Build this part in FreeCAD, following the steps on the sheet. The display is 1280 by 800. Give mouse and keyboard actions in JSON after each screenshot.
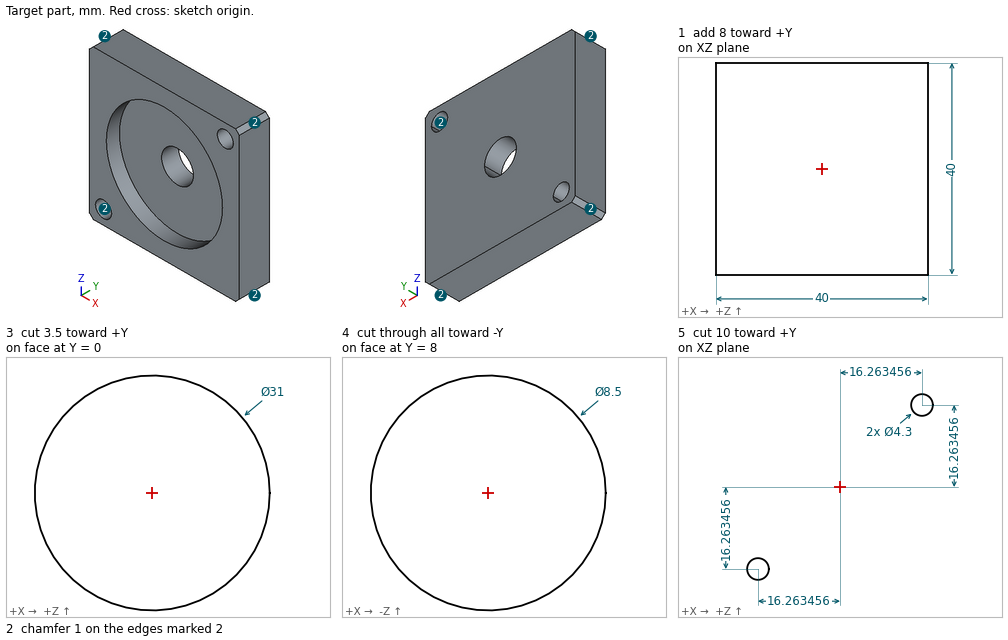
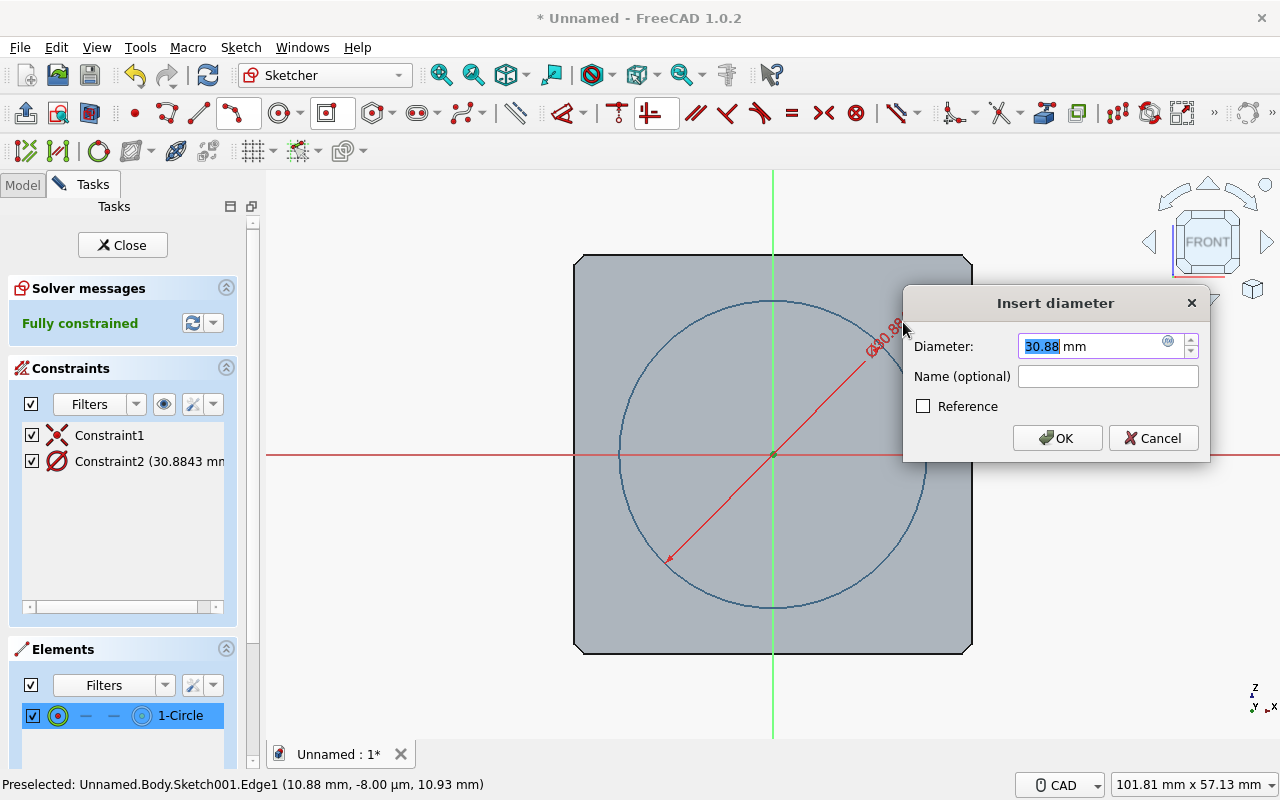
{"action": "type", "text": "31"}
{"action": "key", "text": "Return"}
{"action": "key", "text": "Escape"}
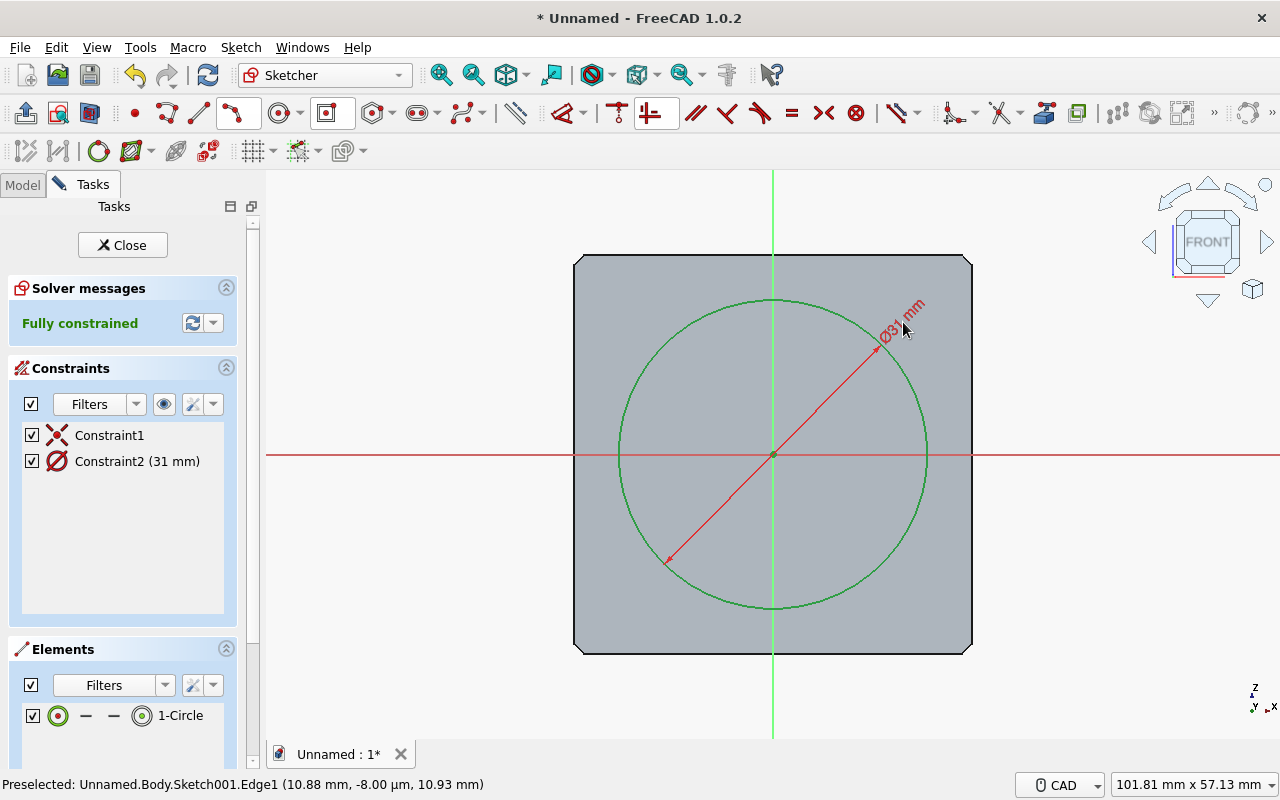
{"action": "left_click", "coordinate": [123, 245]}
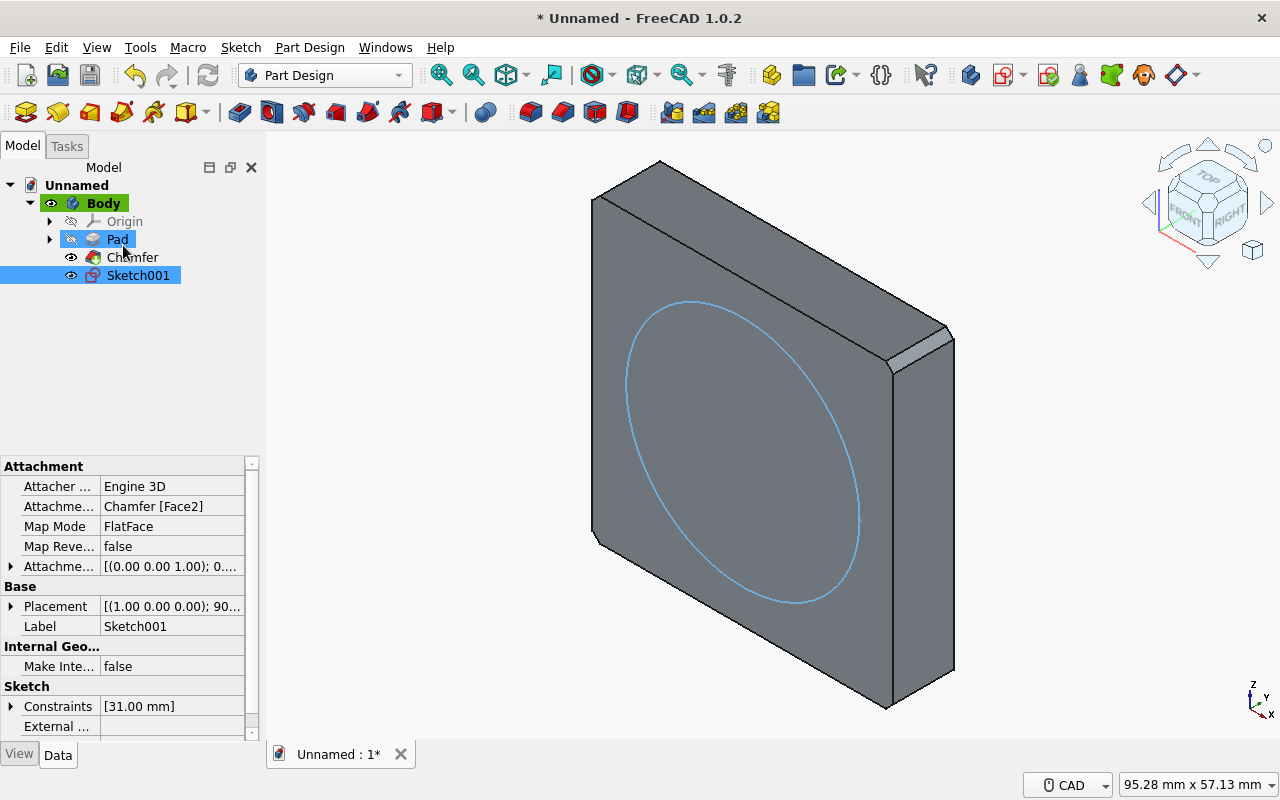
{"action": "left_click", "coordinate": [240, 112]}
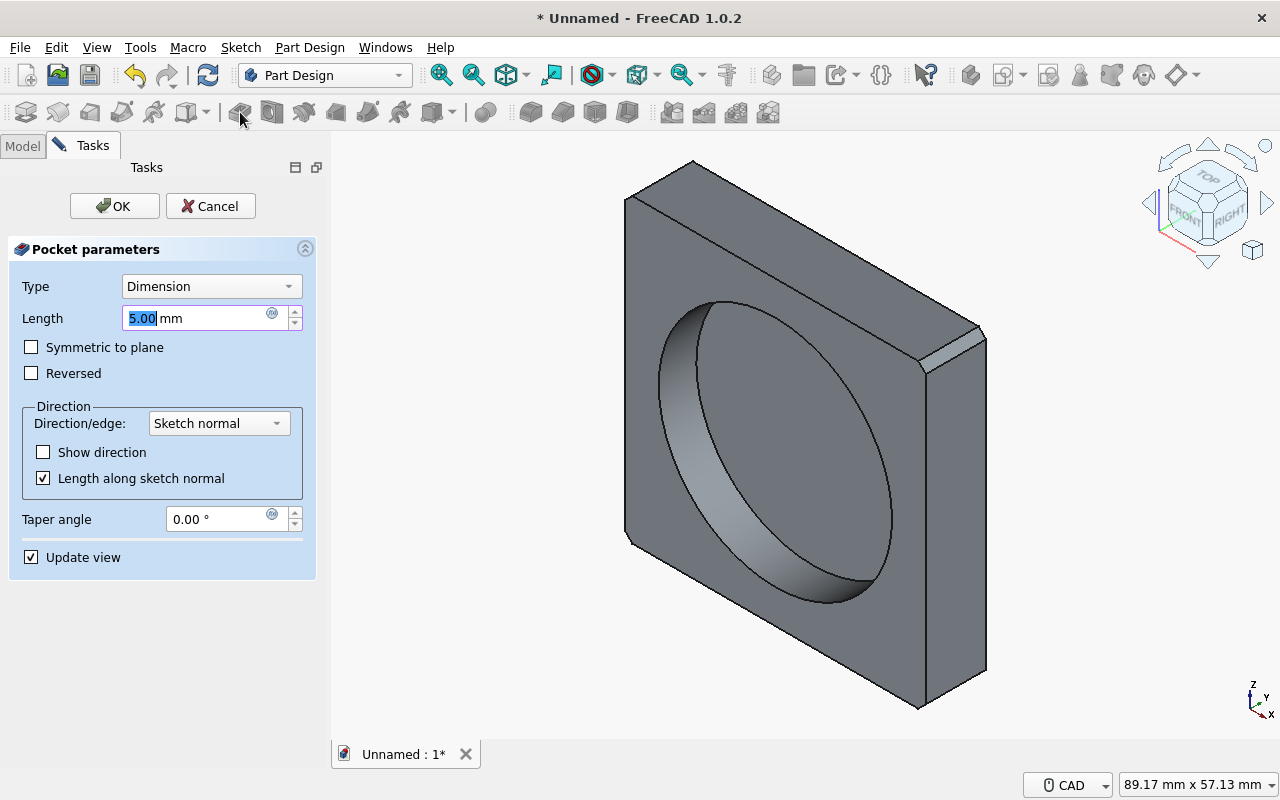
{"action": "type", "text": "3.5"}
{"action": "key", "text": "Tab"}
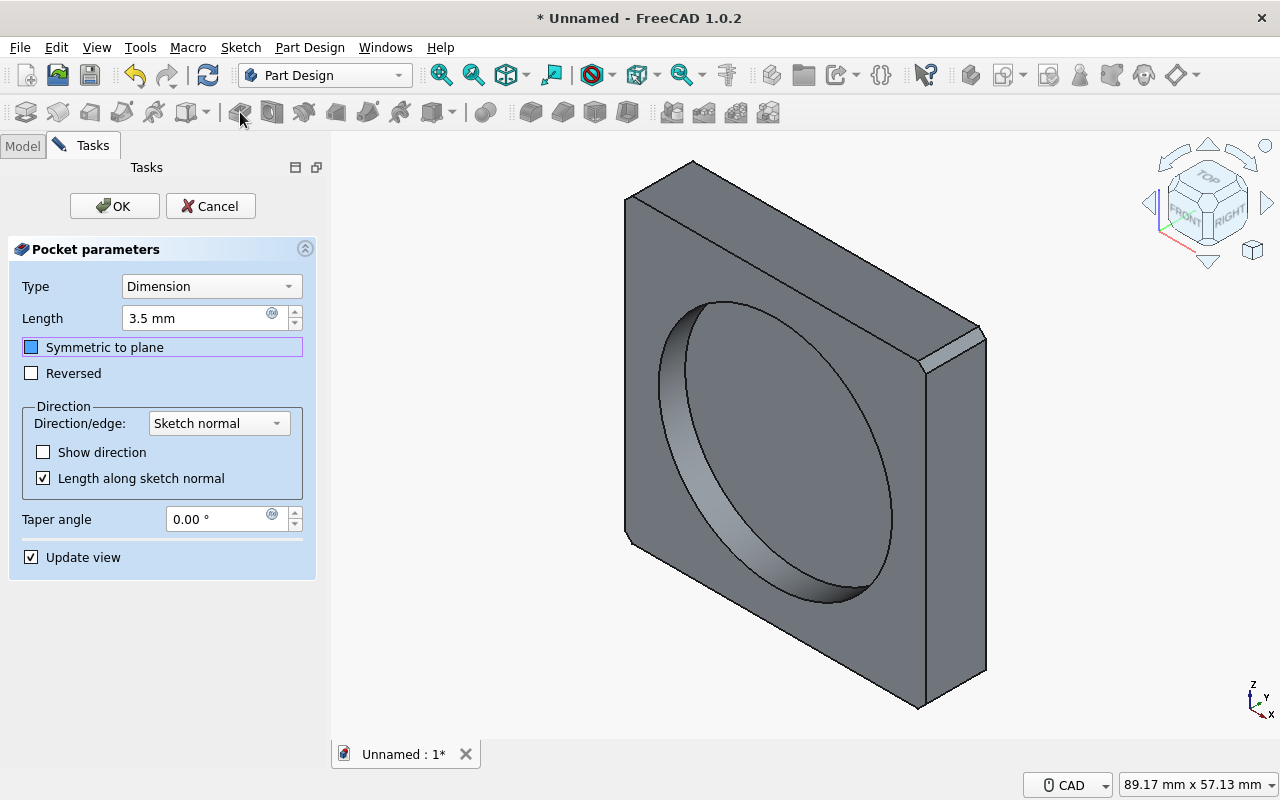
{"action": "left_click", "coordinate": [115, 206]}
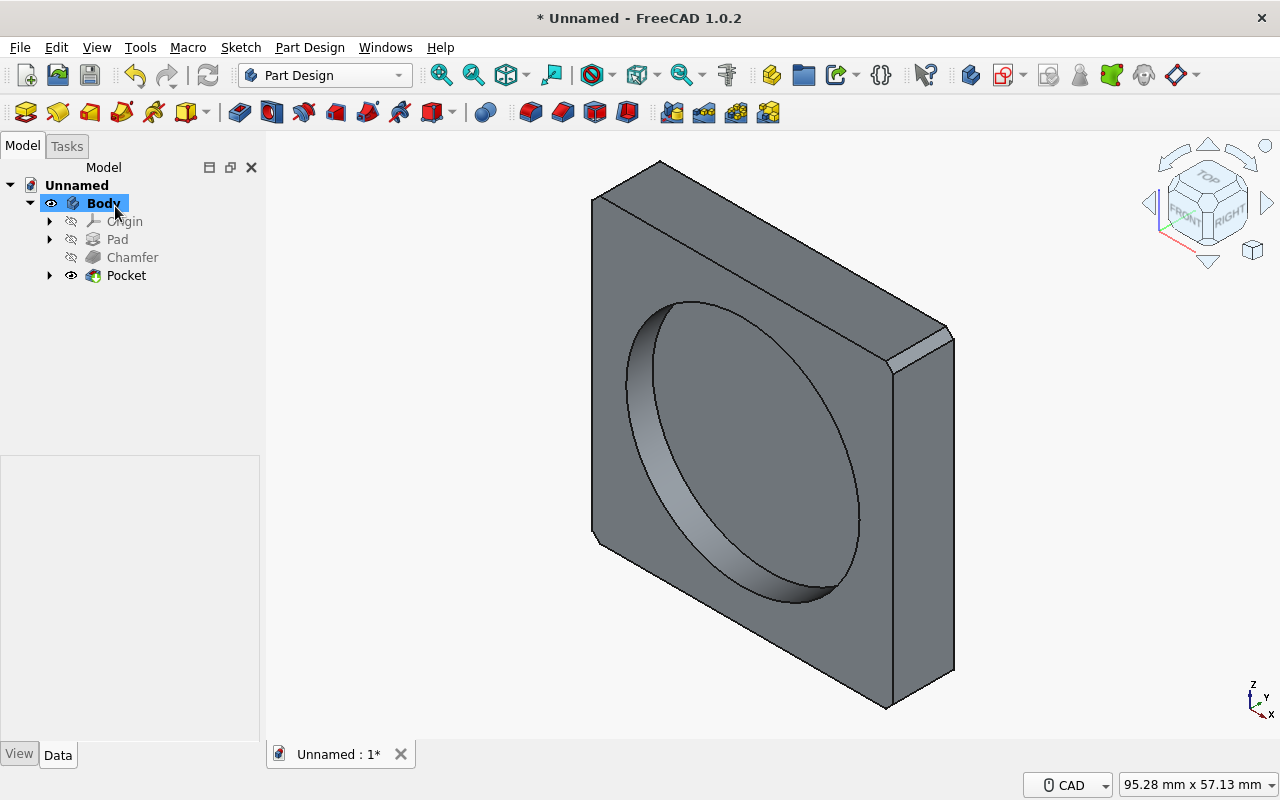
{"action": "key", "text": "4"}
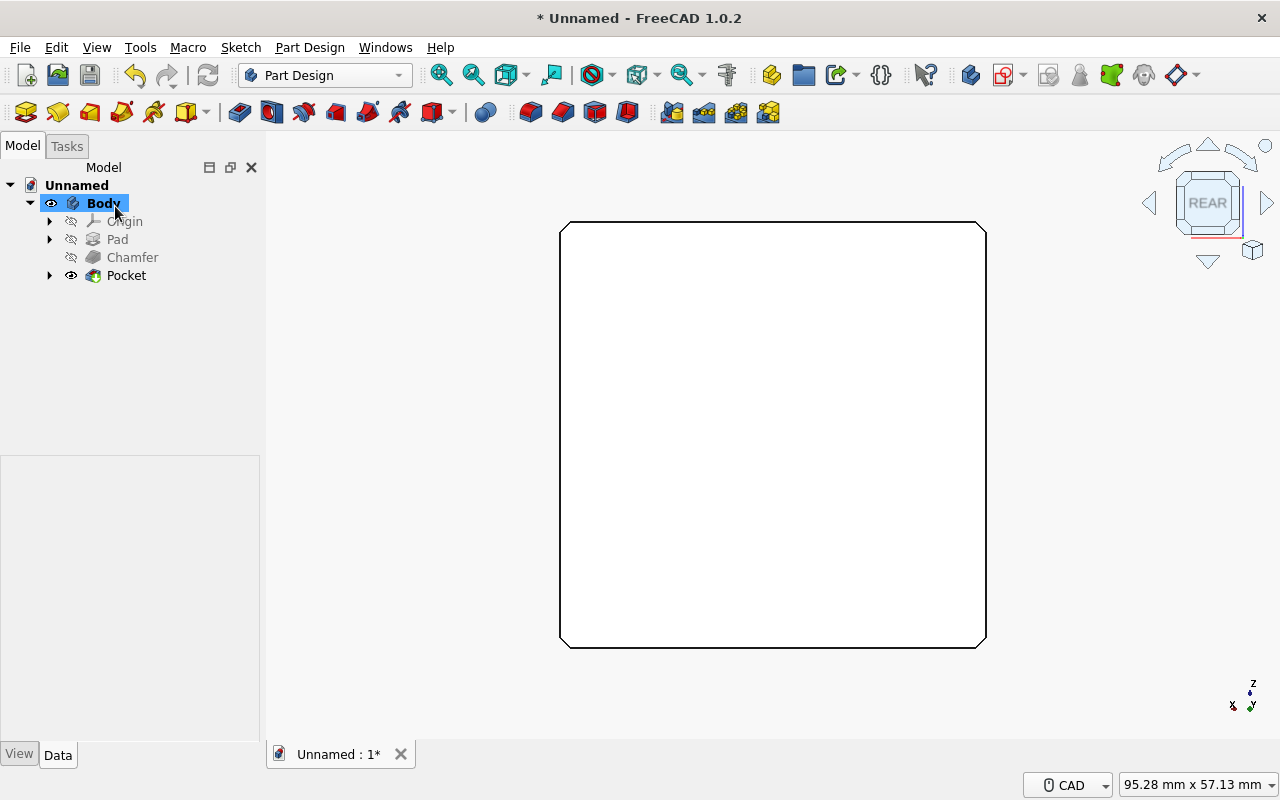
{"action": "left_click", "coordinate": [773, 434]}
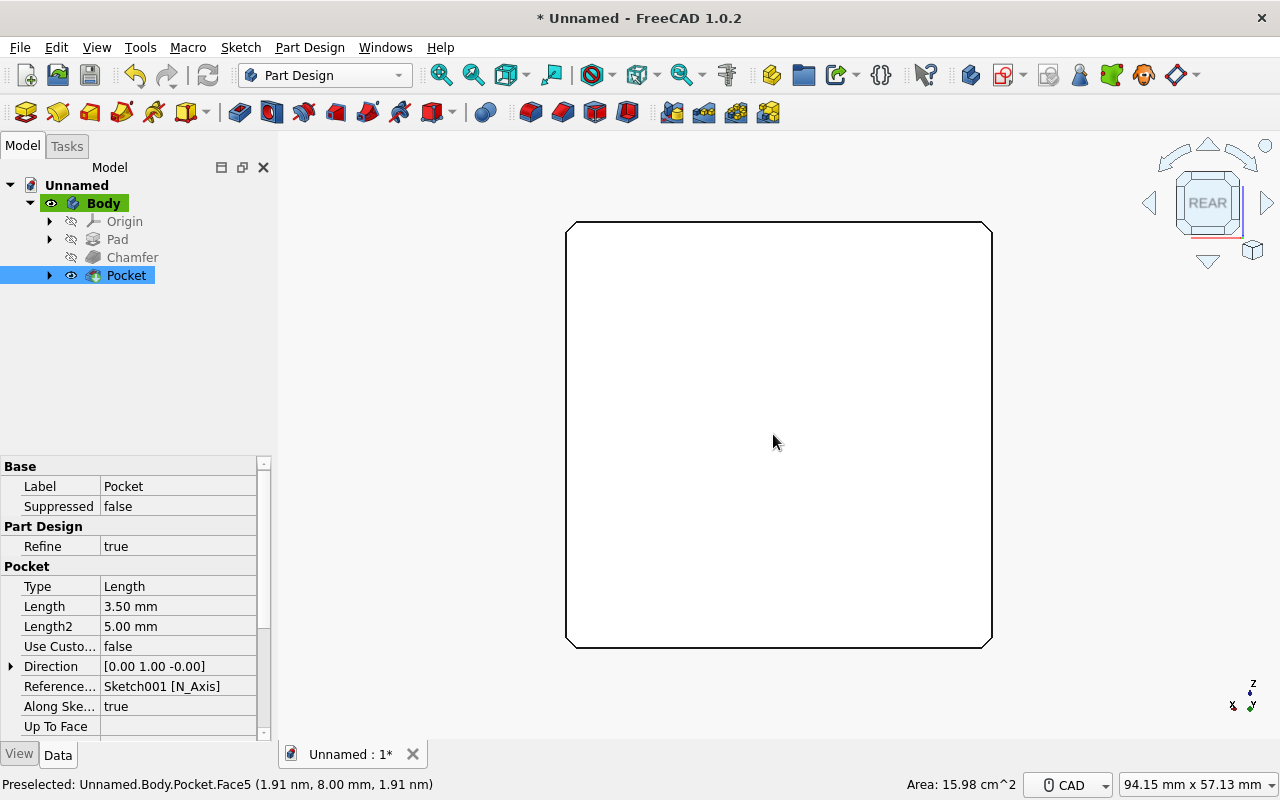
{"action": "left_click", "coordinate": [1004, 76]}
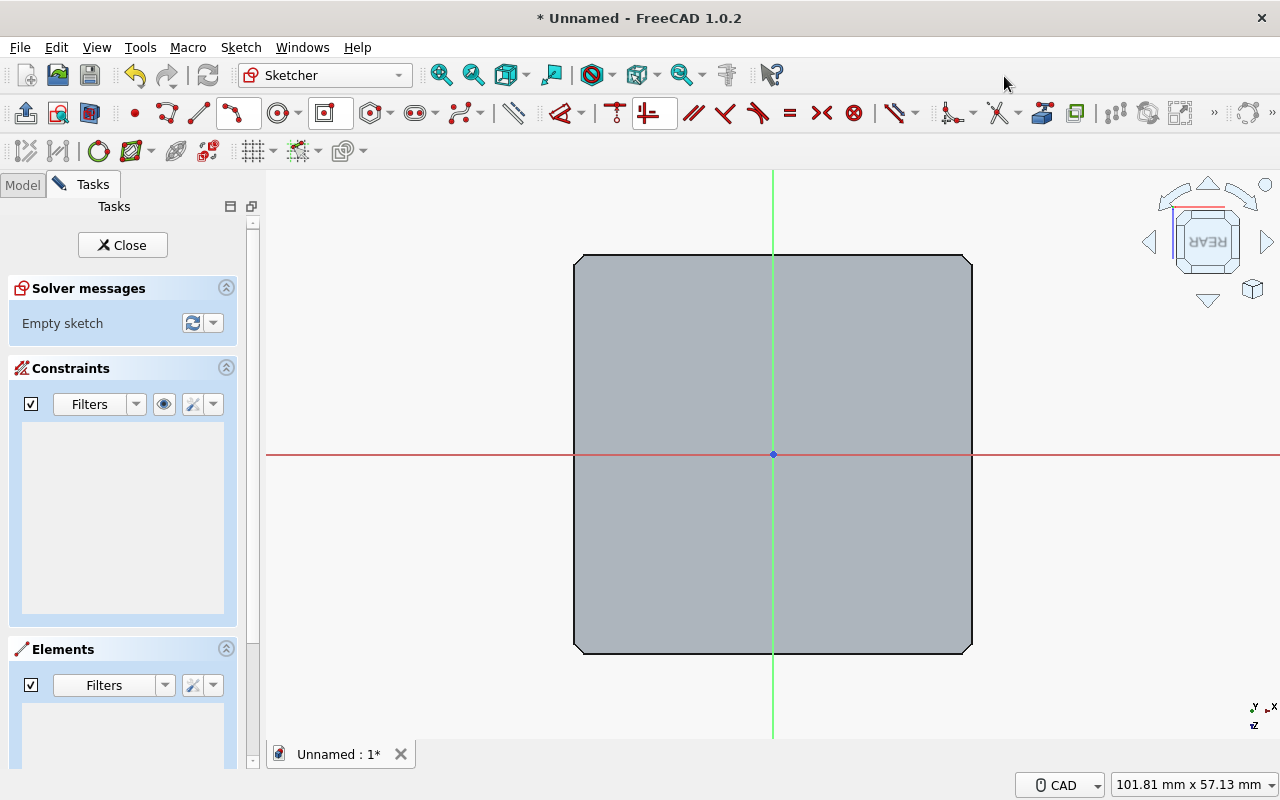
{"action": "scroll", "coordinate": [795, 454], "scroll_direction": "up", "scroll_amount": 7}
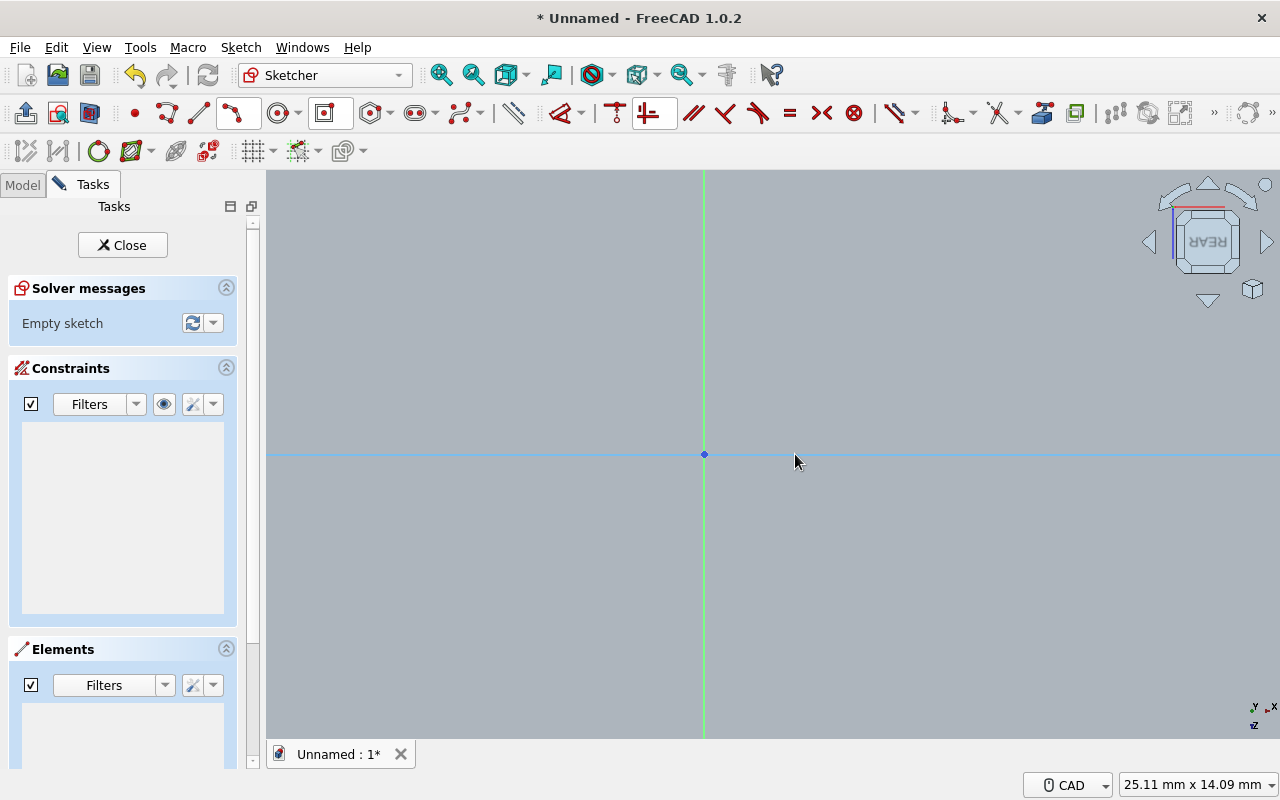
{"action": "left_click", "coordinate": [278, 114]}